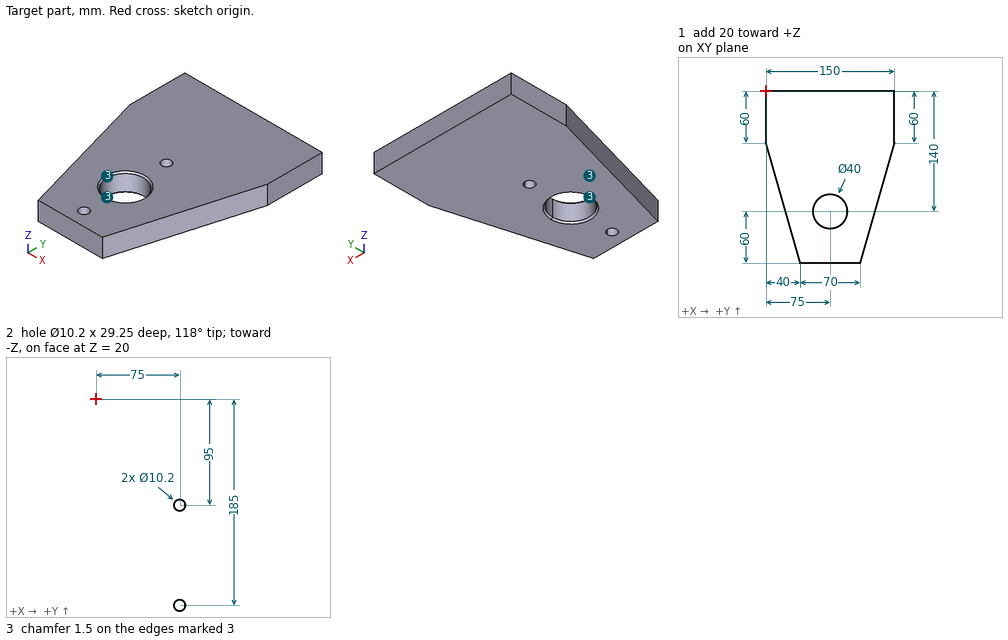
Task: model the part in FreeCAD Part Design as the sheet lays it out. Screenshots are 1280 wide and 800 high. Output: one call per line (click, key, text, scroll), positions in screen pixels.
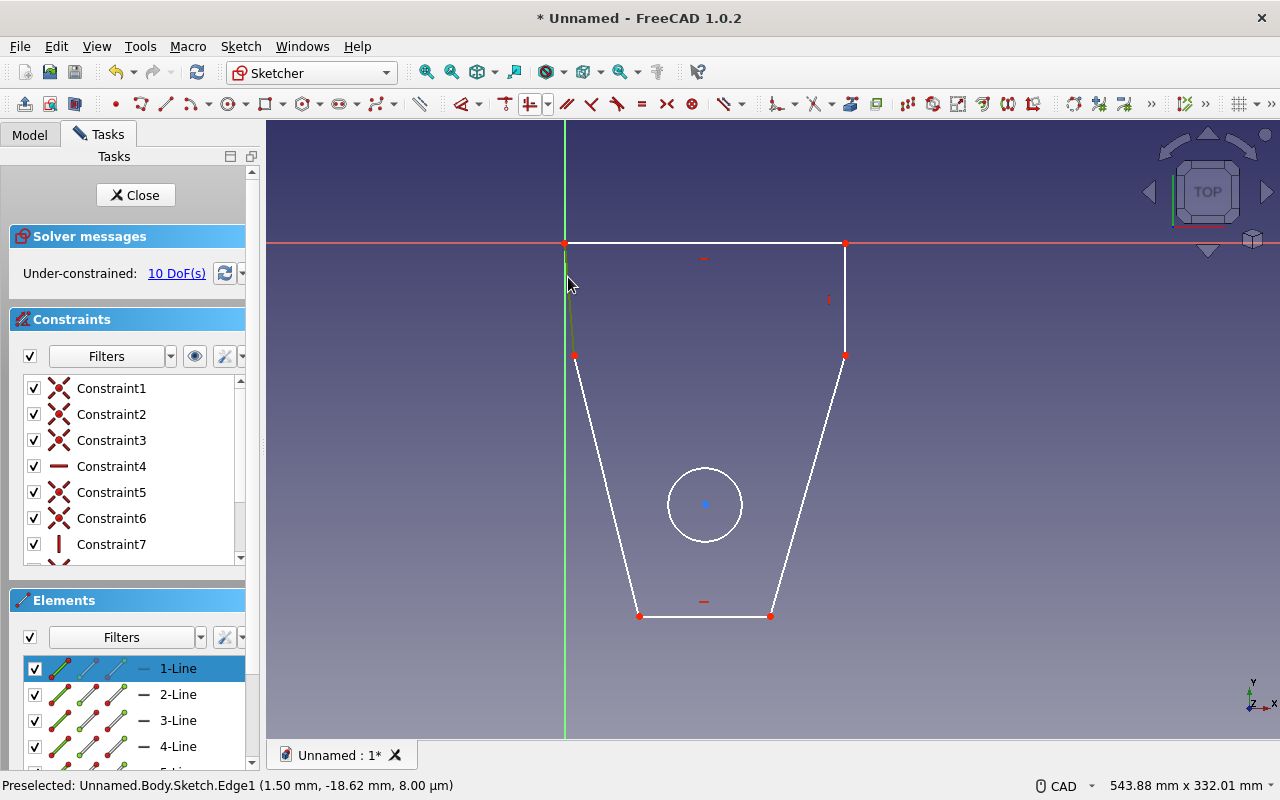
key(v)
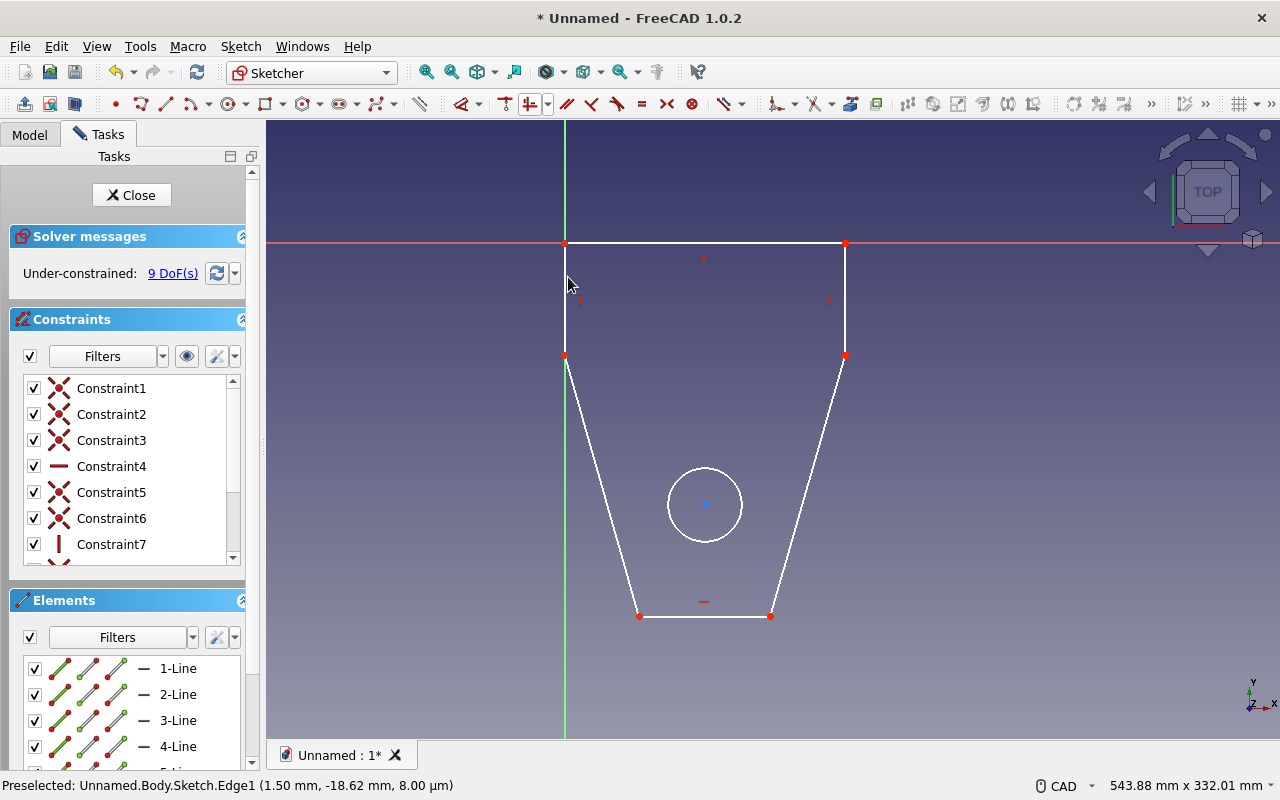
click(731, 479)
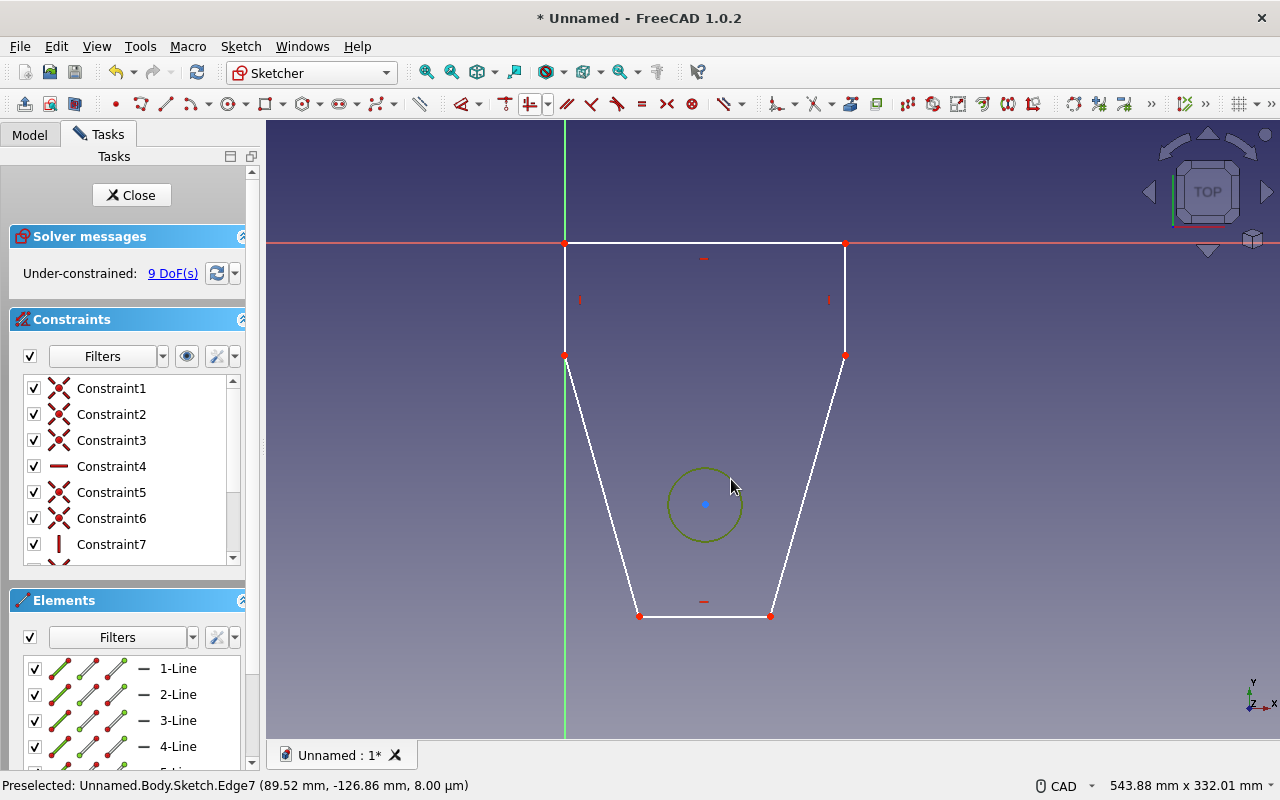
click(478, 104)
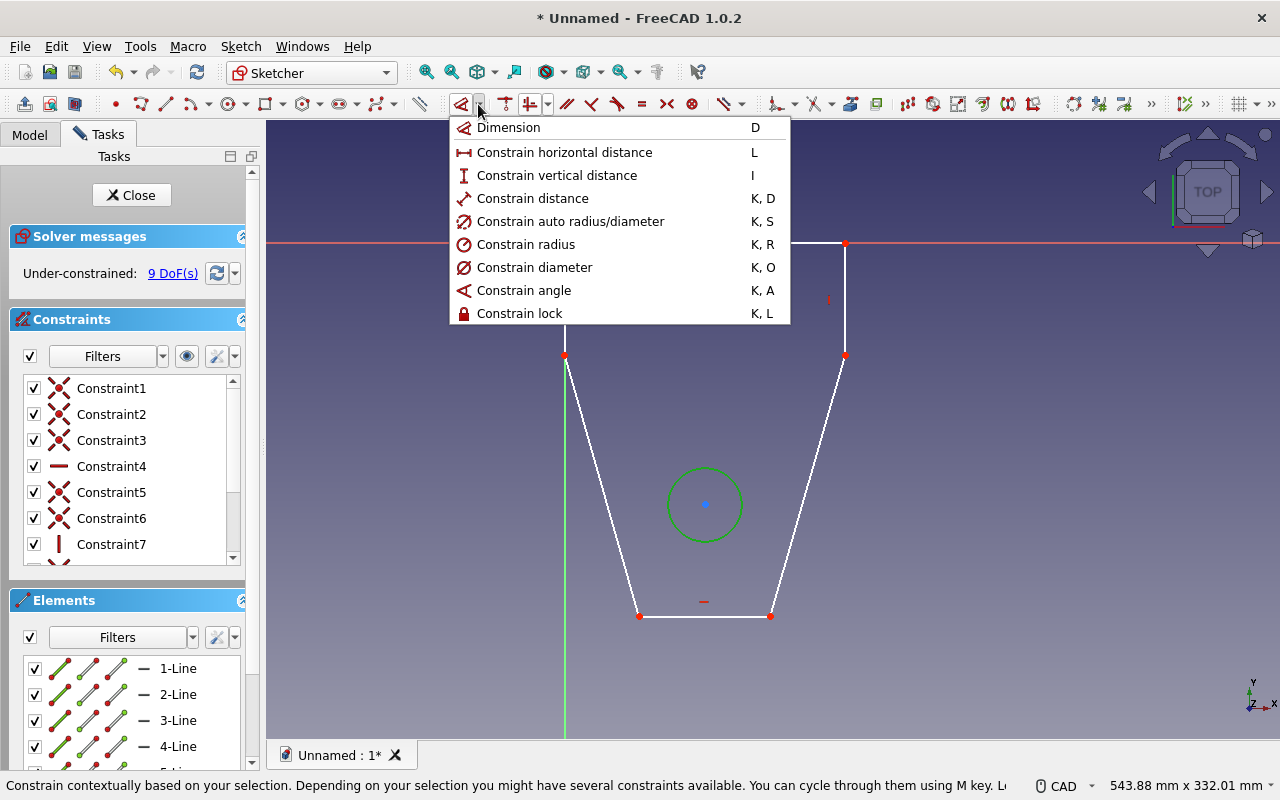
click(620, 268)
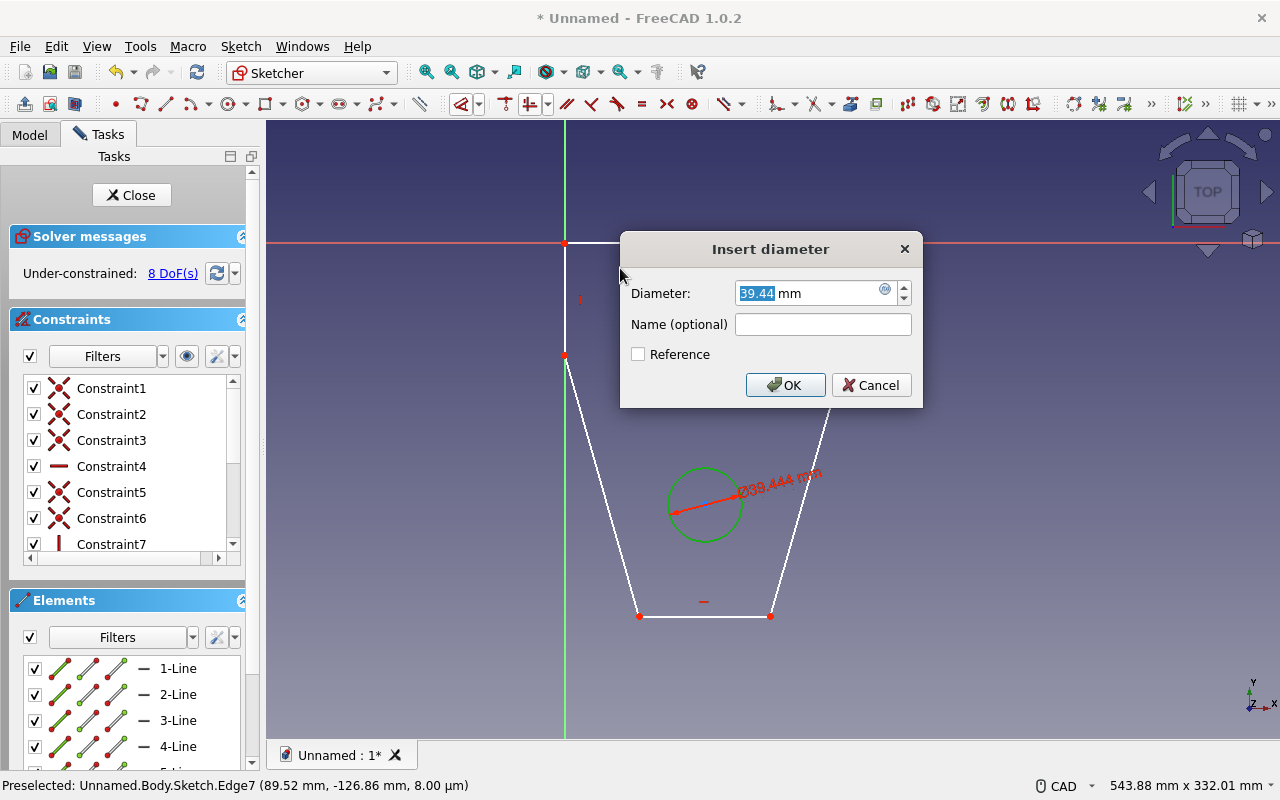
text(40)
key(Return)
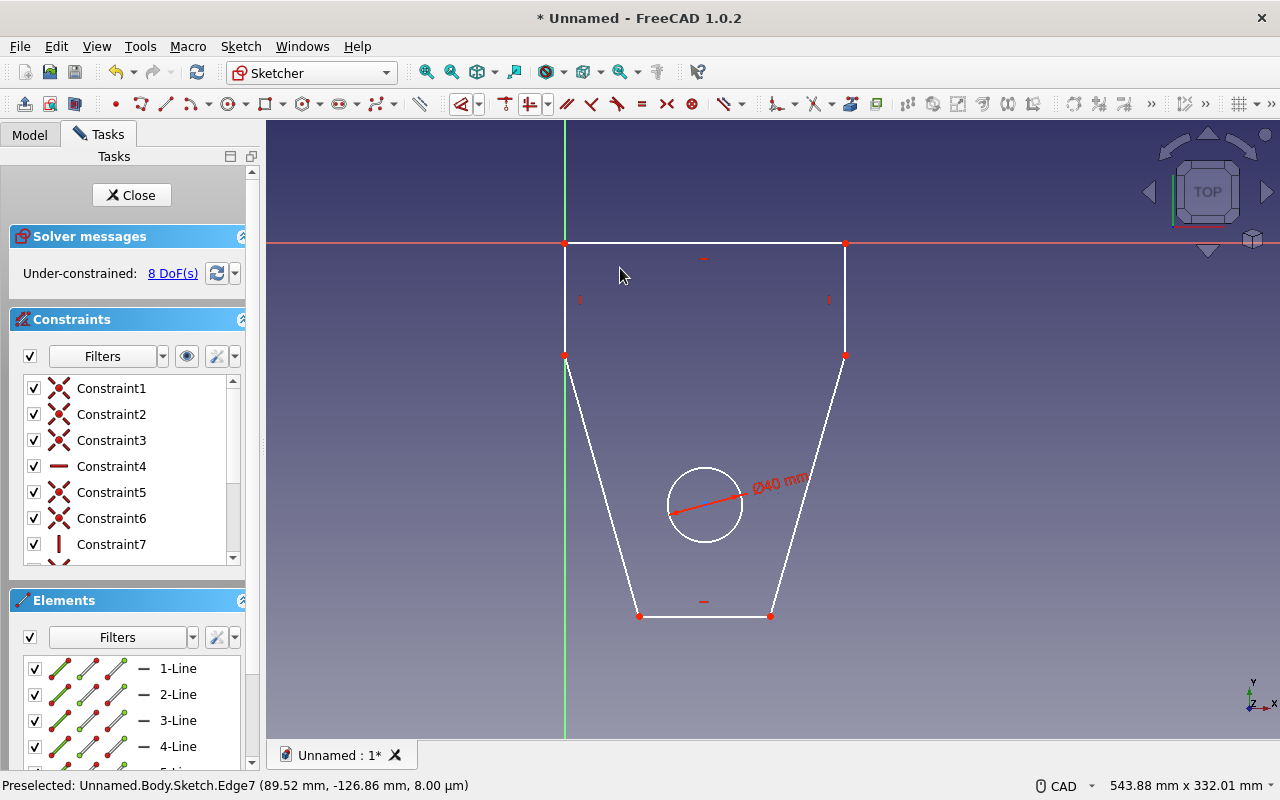
click(565, 277)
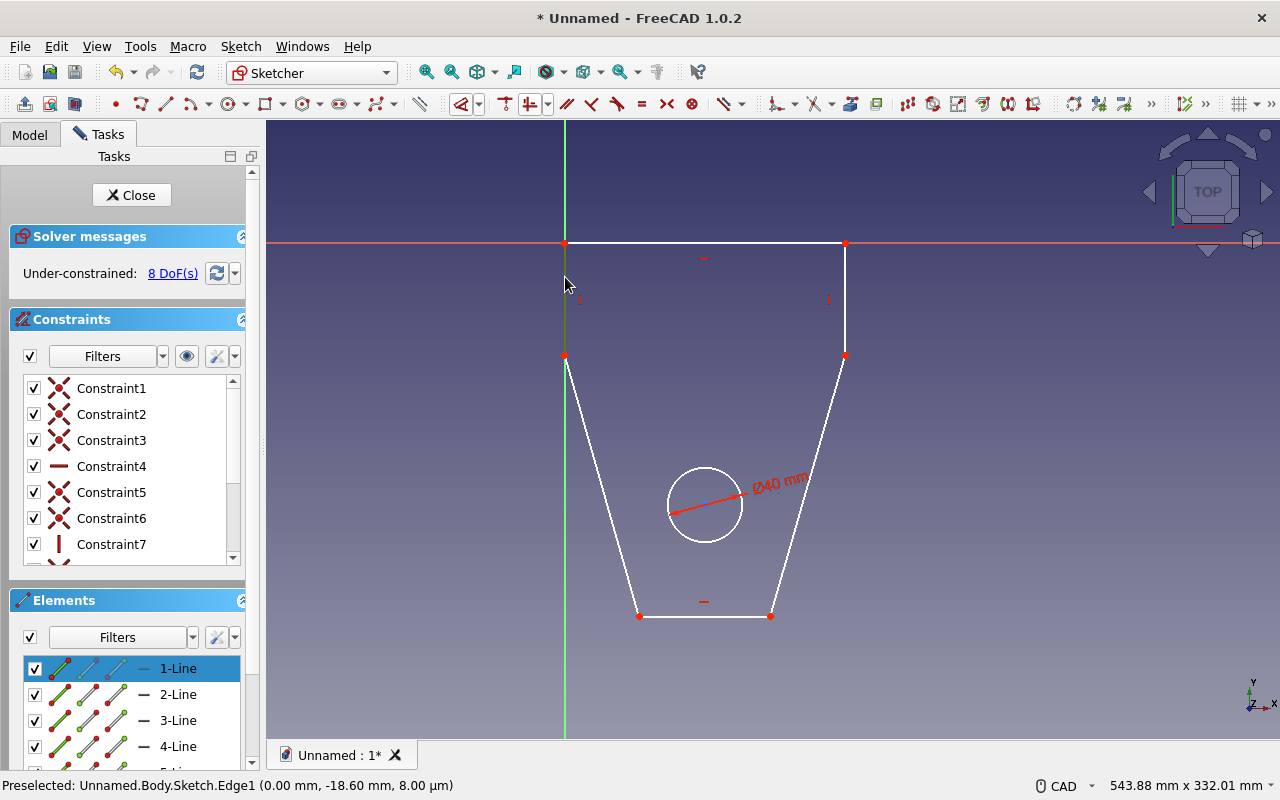
click(478, 104)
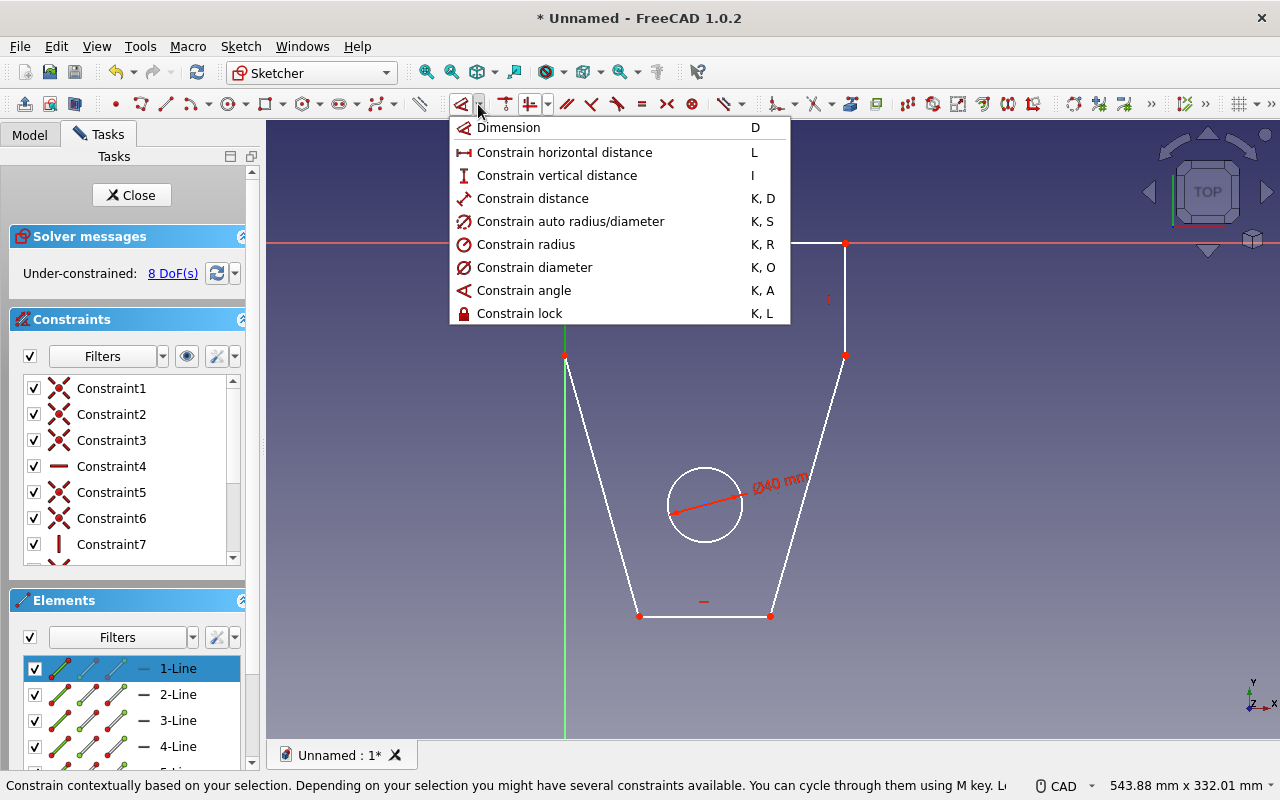
click(620, 176)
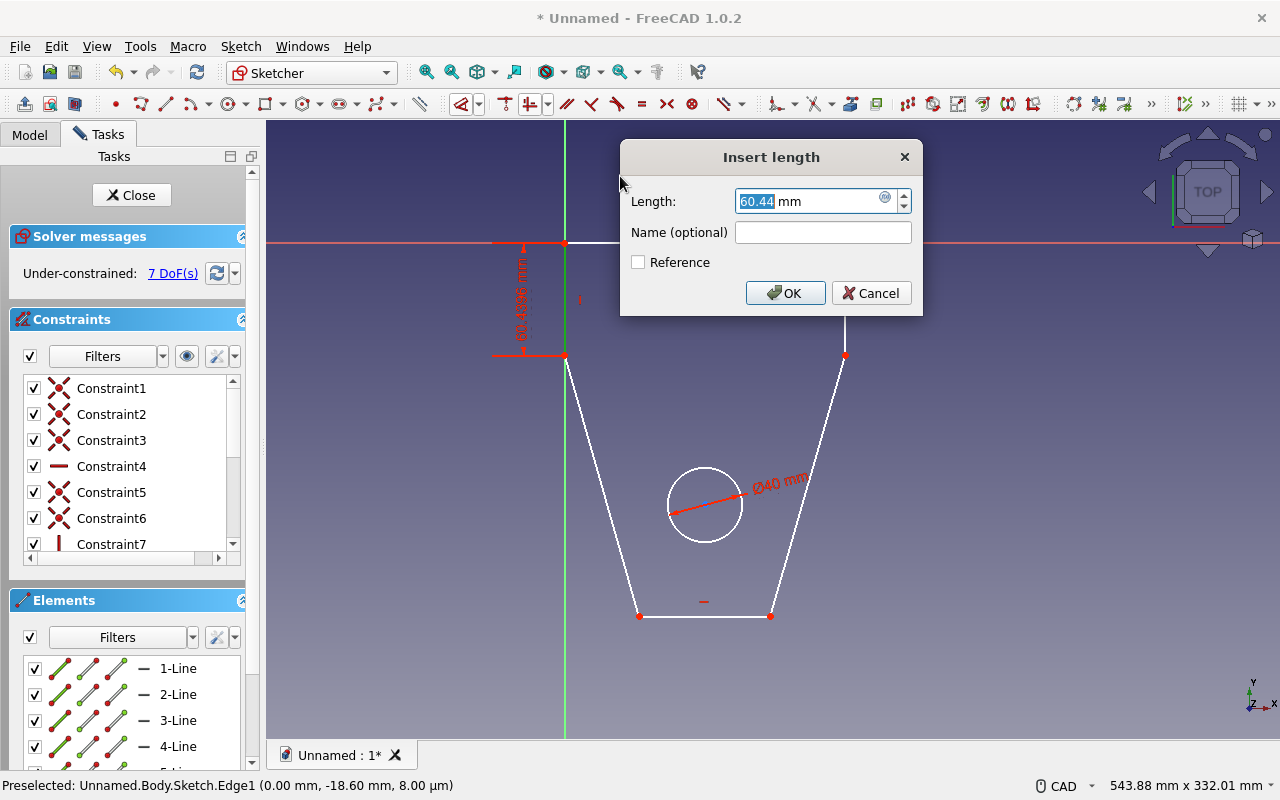
text(60)
key(Return)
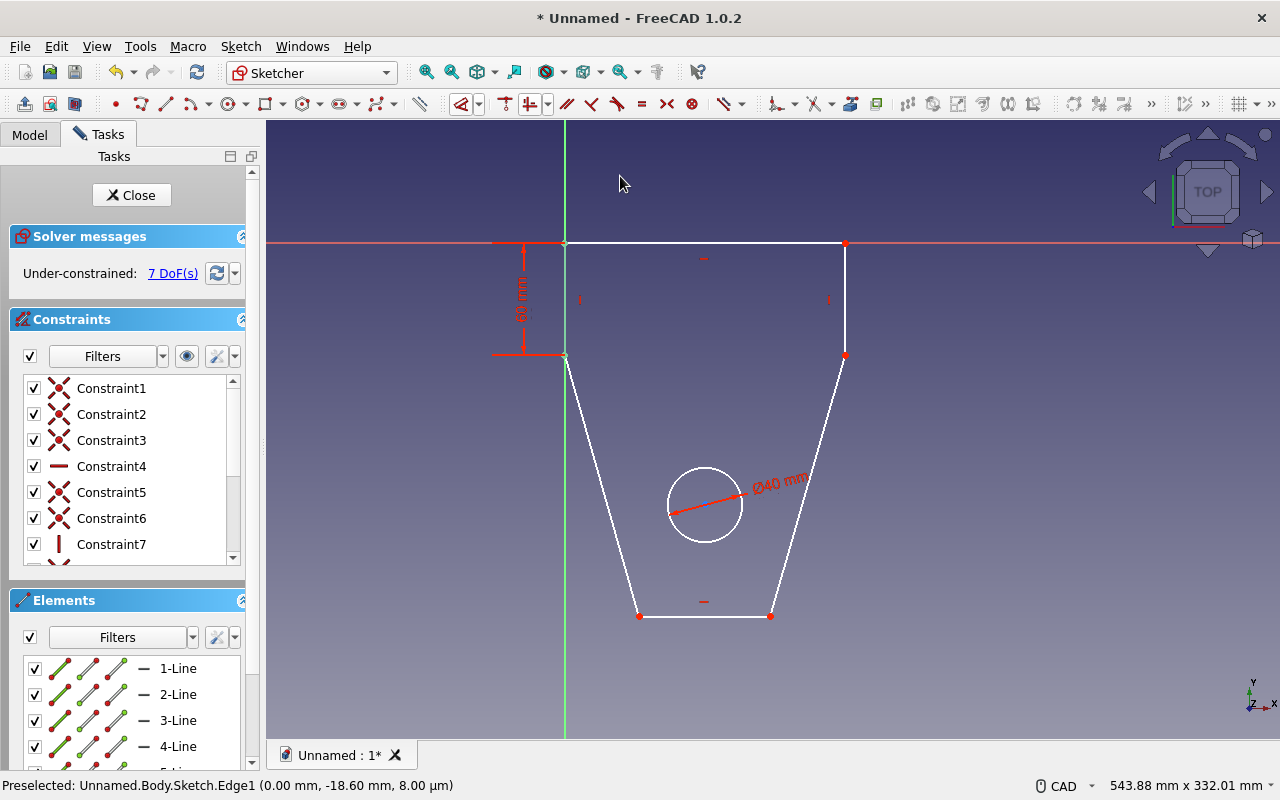
click(678, 617)